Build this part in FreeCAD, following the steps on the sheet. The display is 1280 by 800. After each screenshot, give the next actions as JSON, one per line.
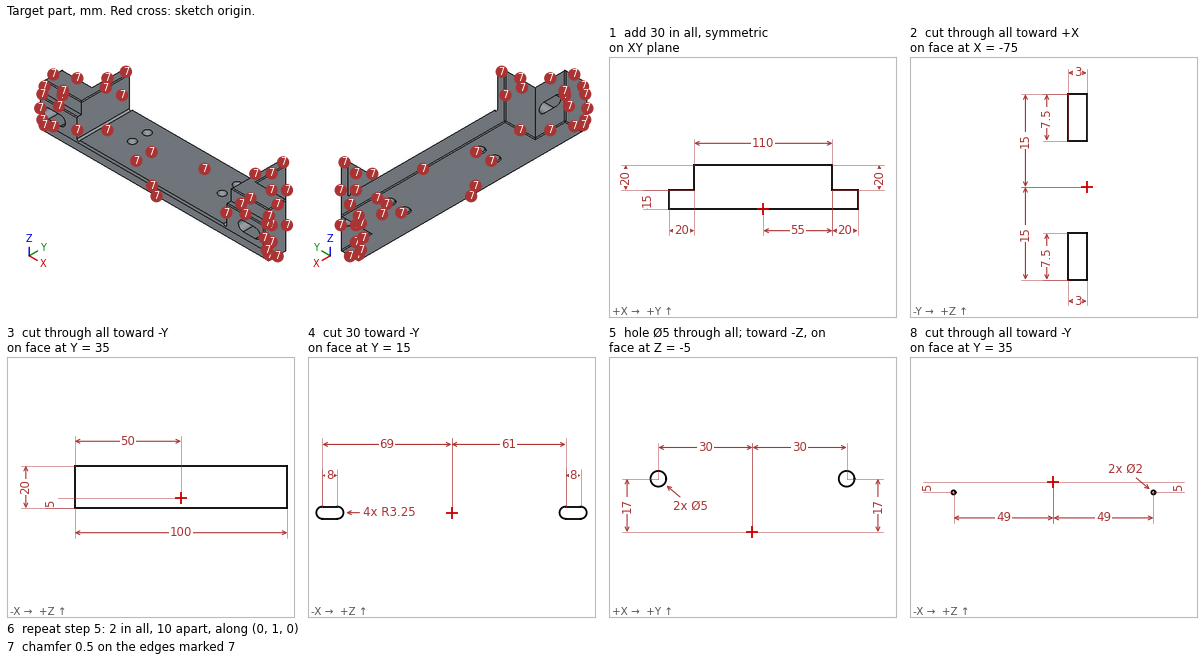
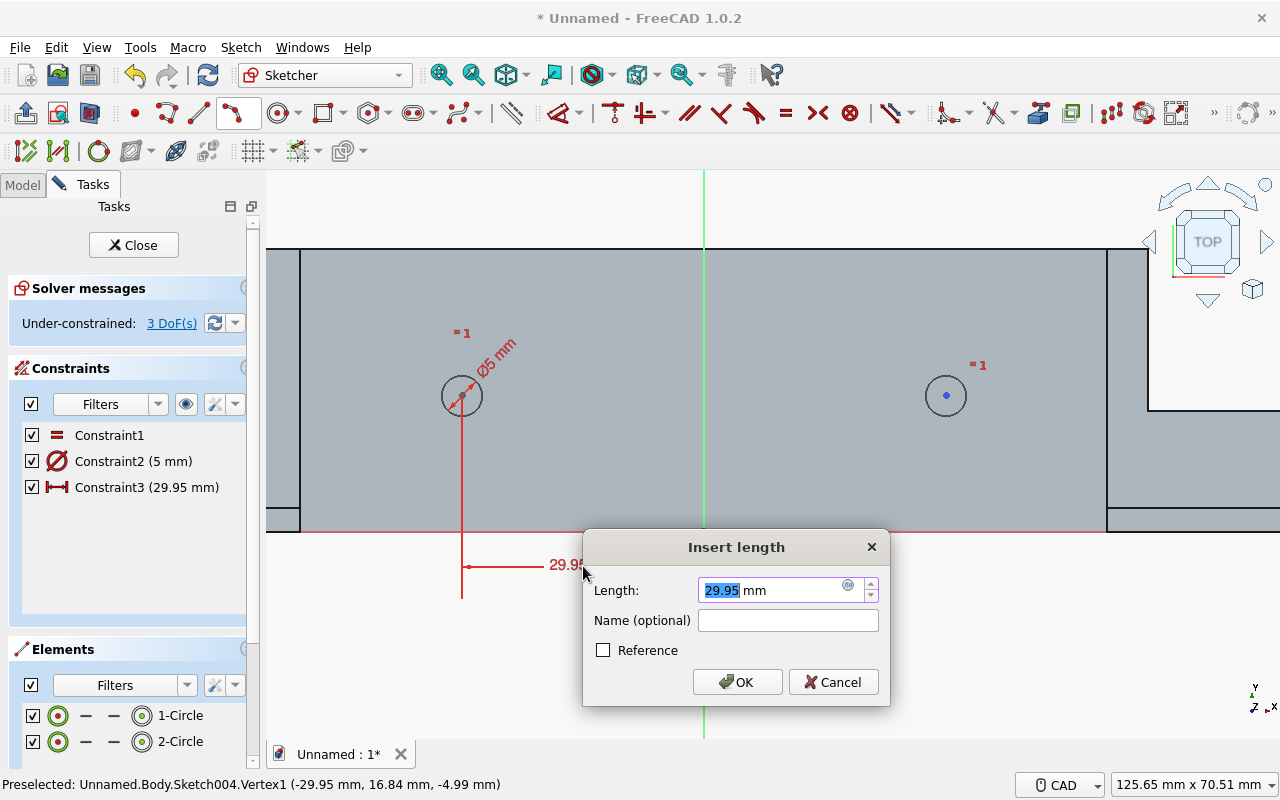
{"action": "type", "text": "30"}
{"action": "key", "text": "Return"}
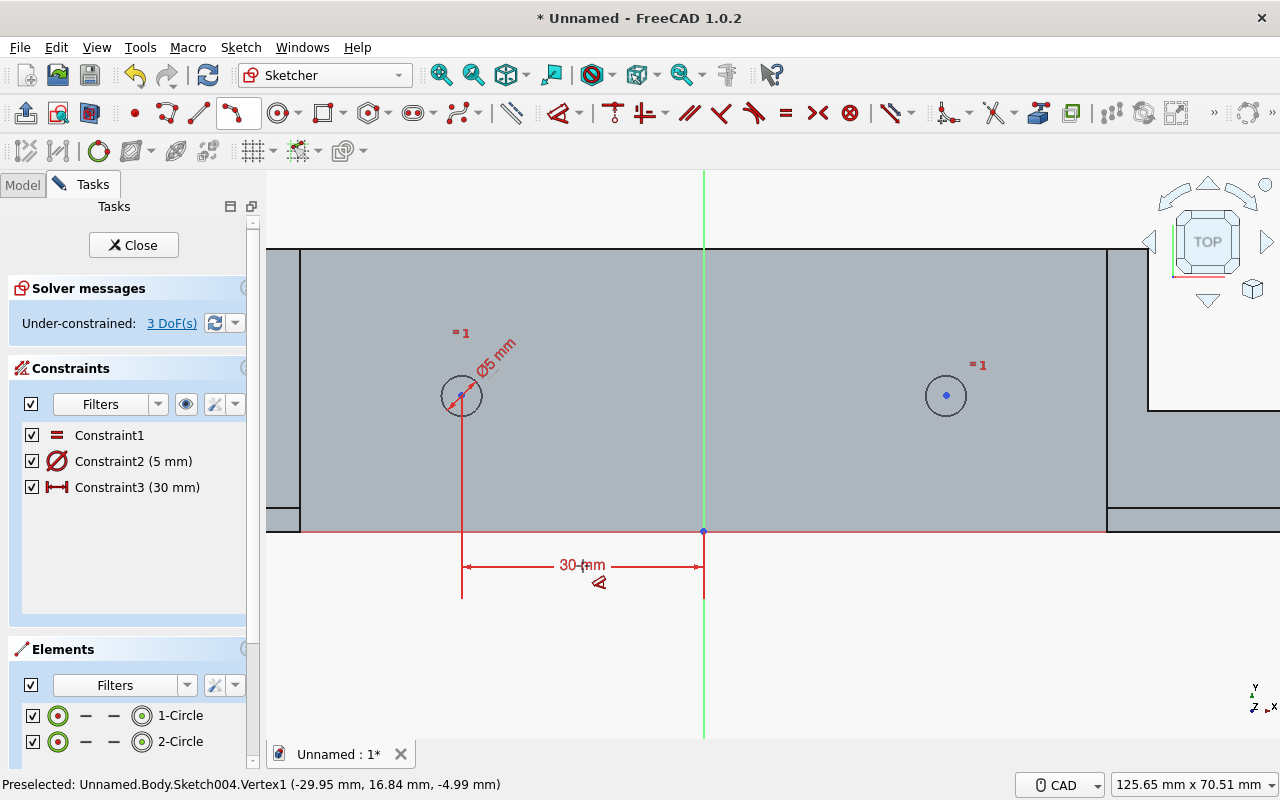
{"action": "left_click", "coordinate": [462, 396]}
{"action": "left_click", "coordinate": [428, 464]}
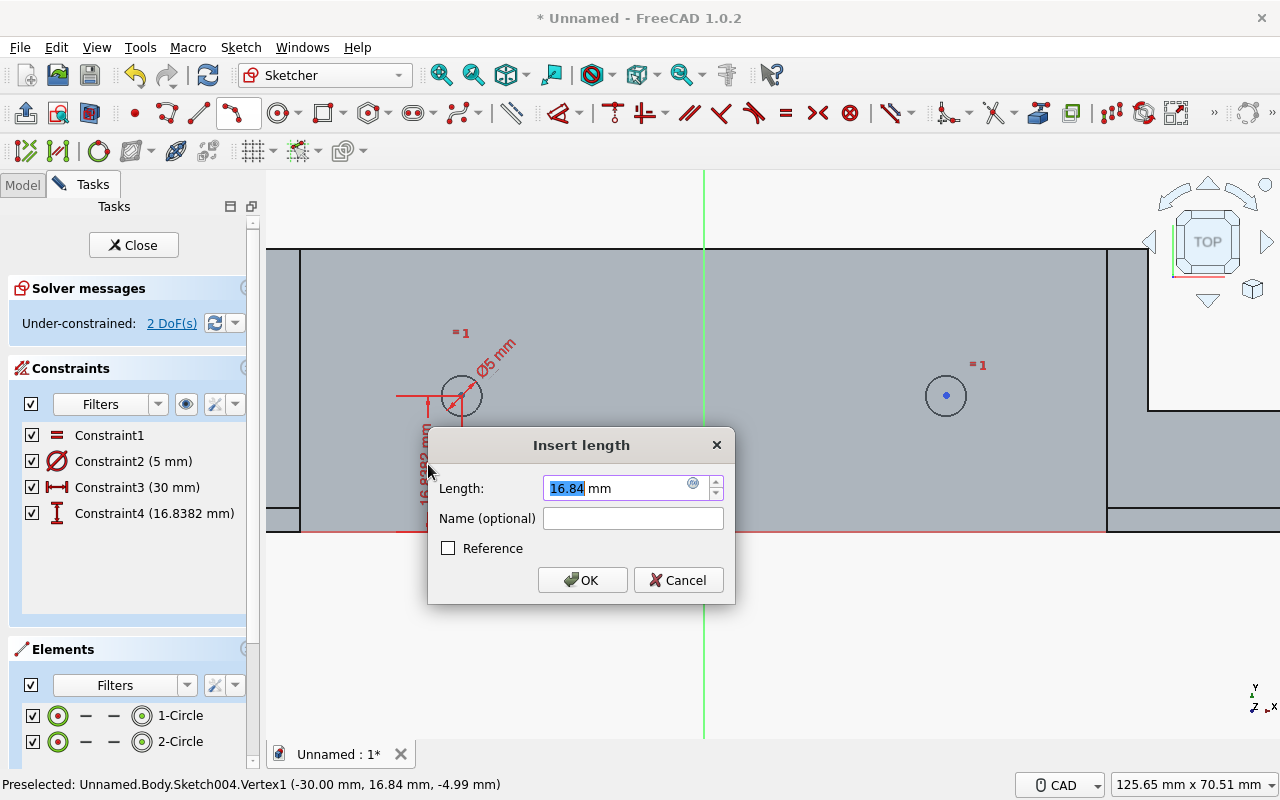
{"action": "type", "text": "17"}
{"action": "key", "text": "Return"}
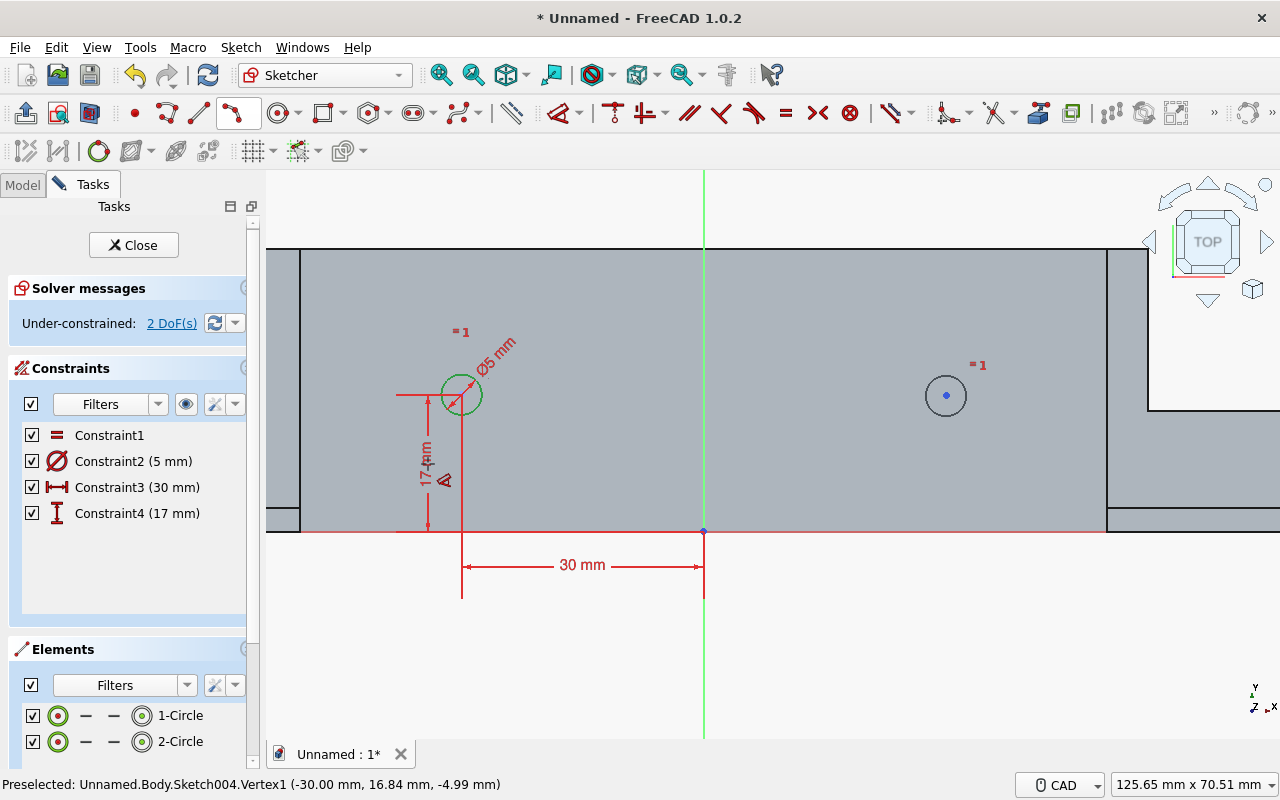
{"action": "left_click", "coordinate": [946, 396]}
{"action": "left_click", "coordinate": [825, 566]}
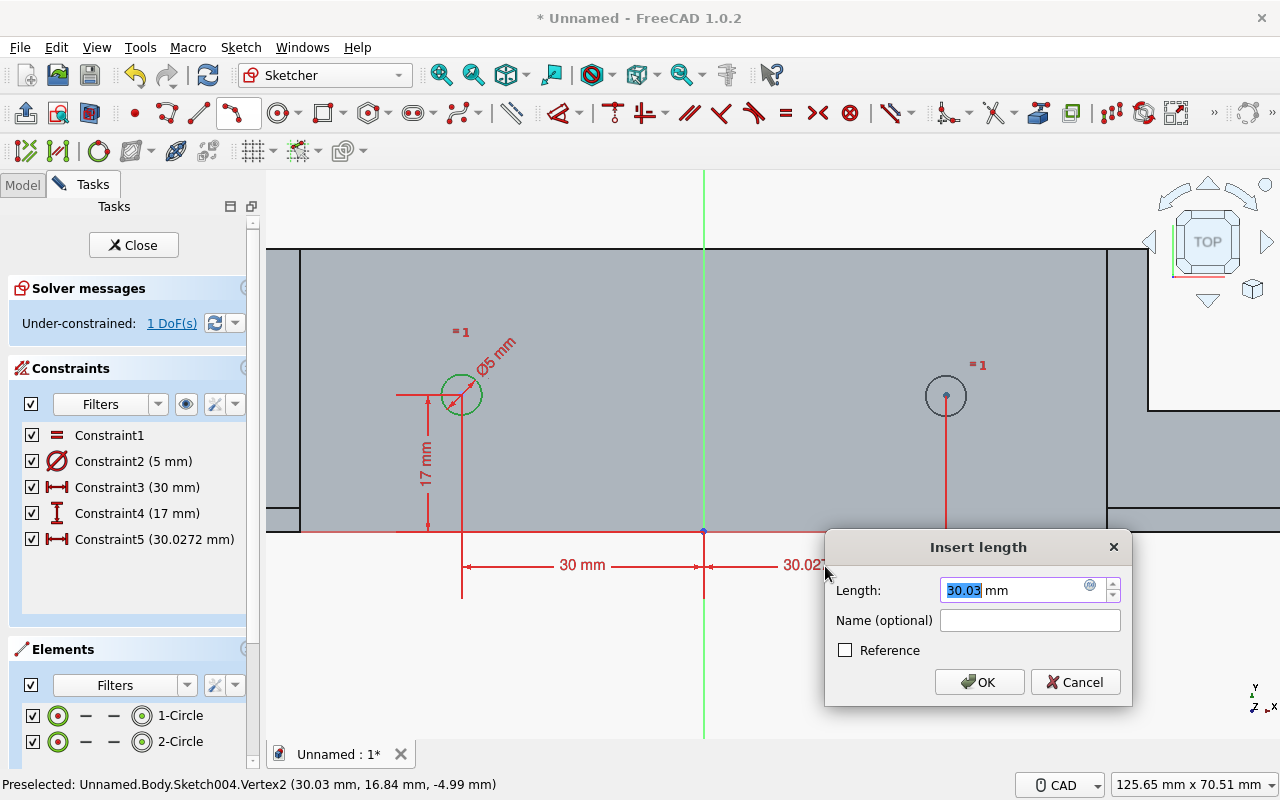
{"action": "type", "text": "30"}
{"action": "key", "text": "Return"}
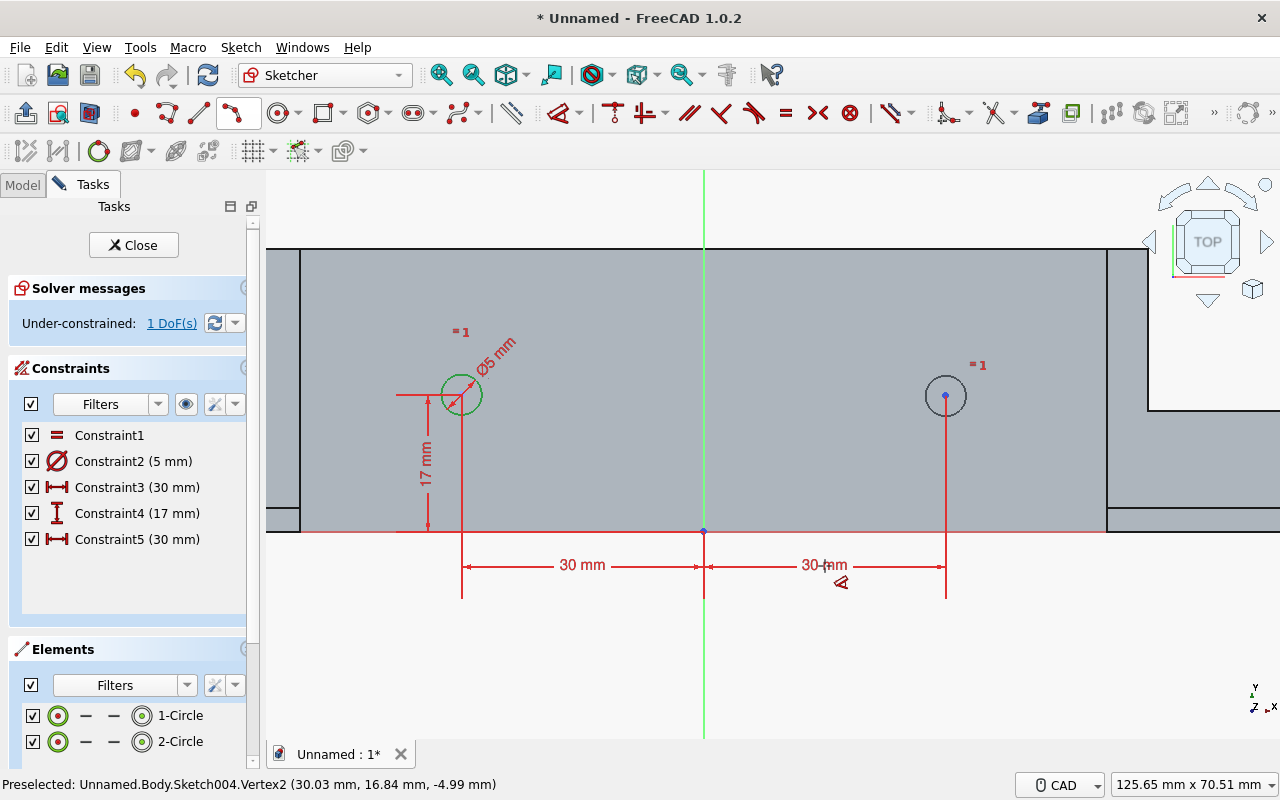
{"action": "left_click", "coordinate": [946, 396]}
{"action": "left_click", "coordinate": [980, 464]}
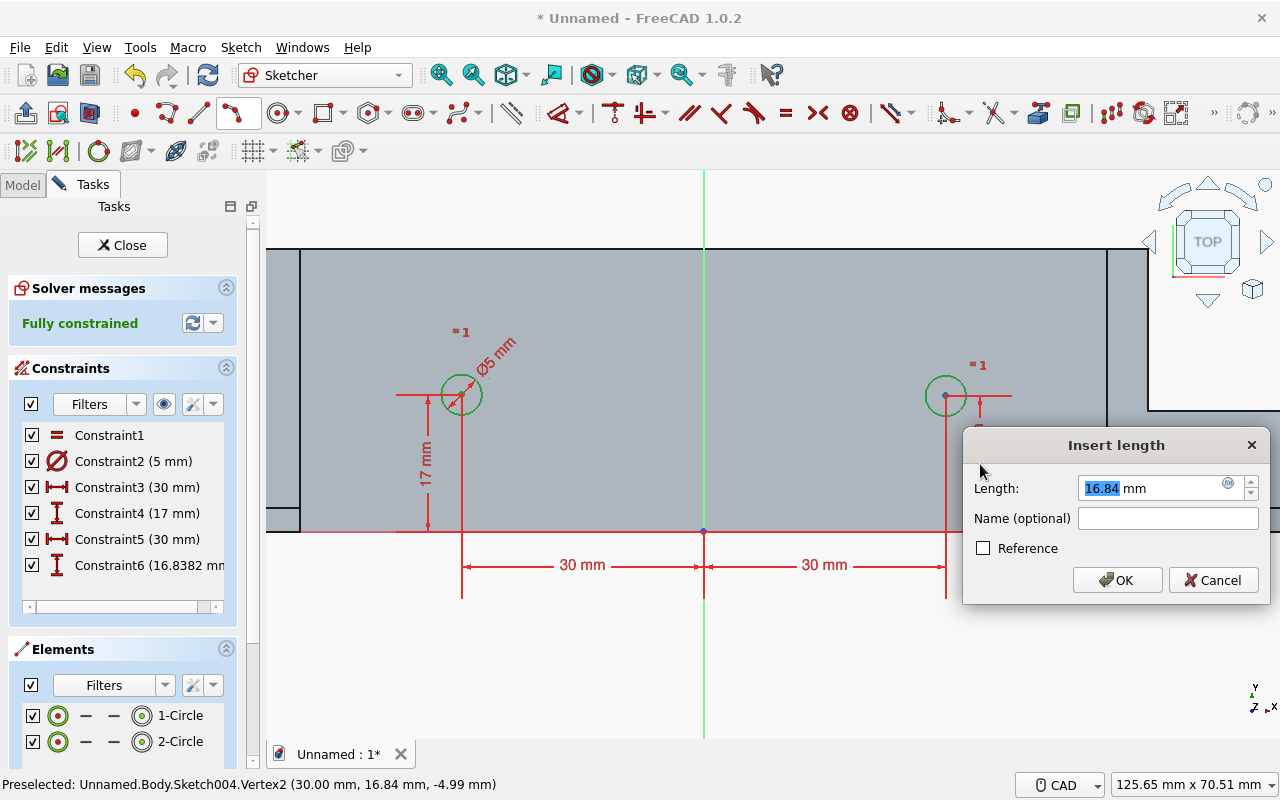
{"action": "type", "text": "17"}
{"action": "key", "text": "Return"}
{"action": "key", "text": "Escape"}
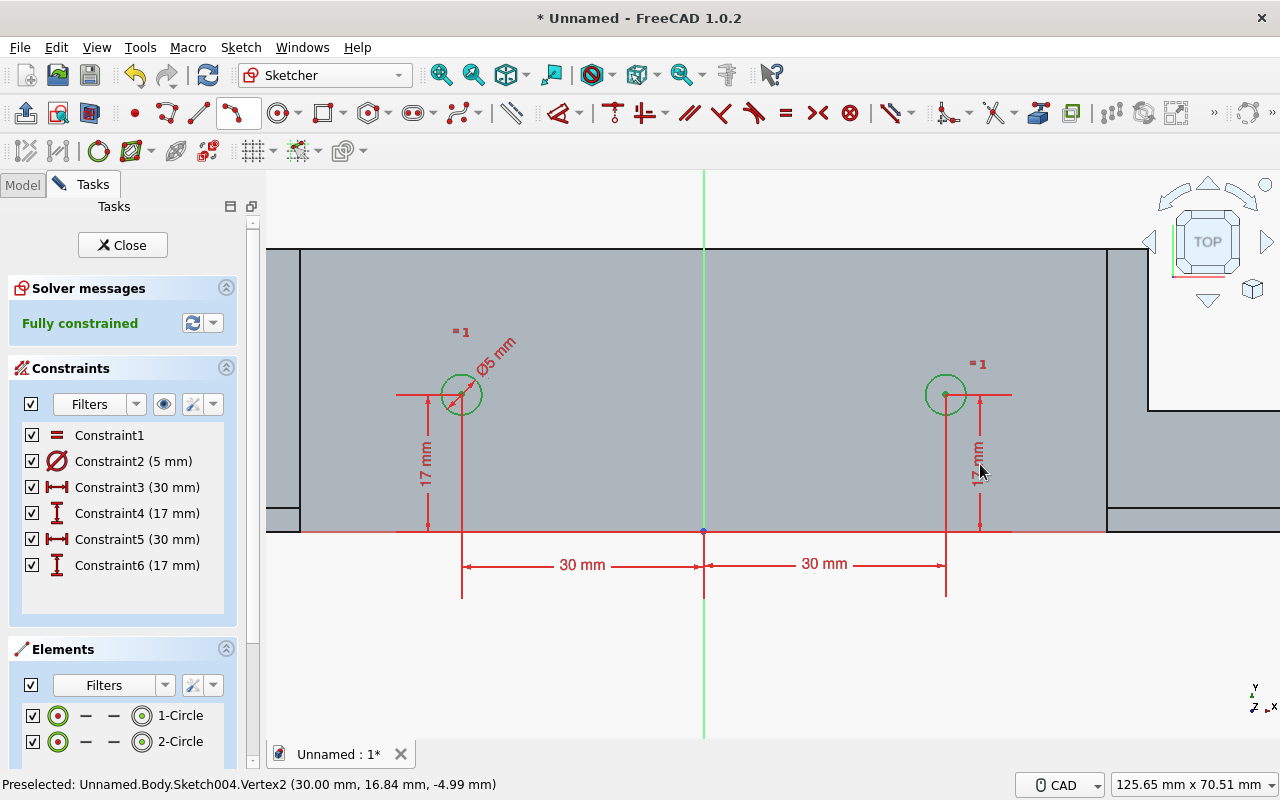
{"action": "left_click", "coordinate": [123, 245]}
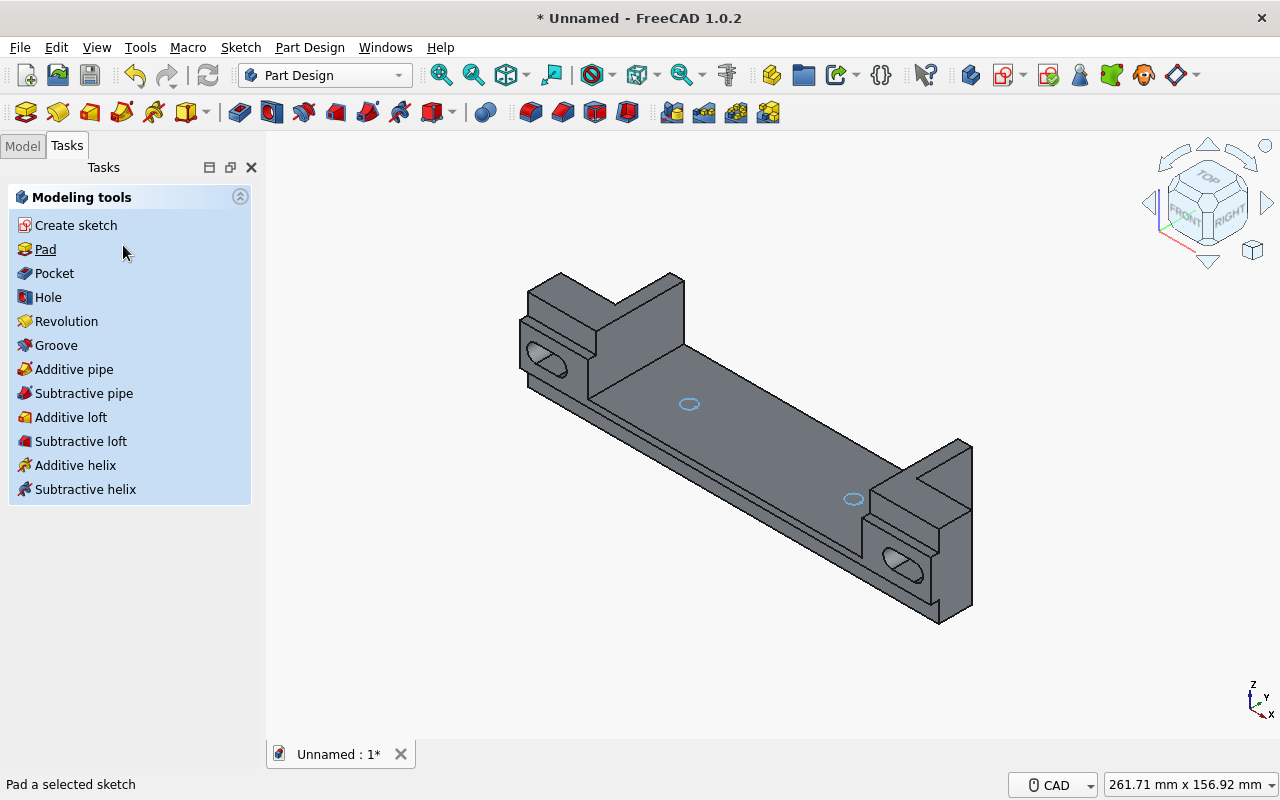
{"action": "left_click", "coordinate": [272, 112]}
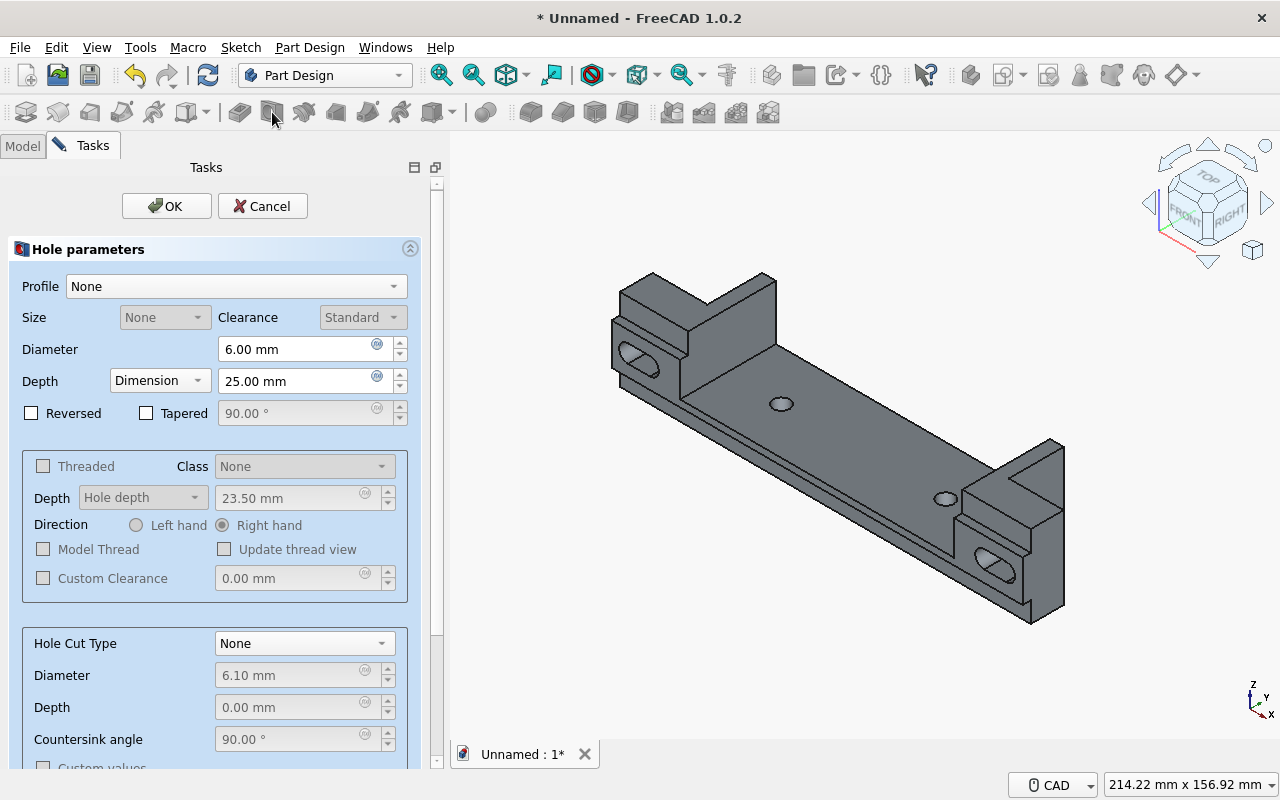
{"action": "triple_click", "coordinate": [305, 349]}